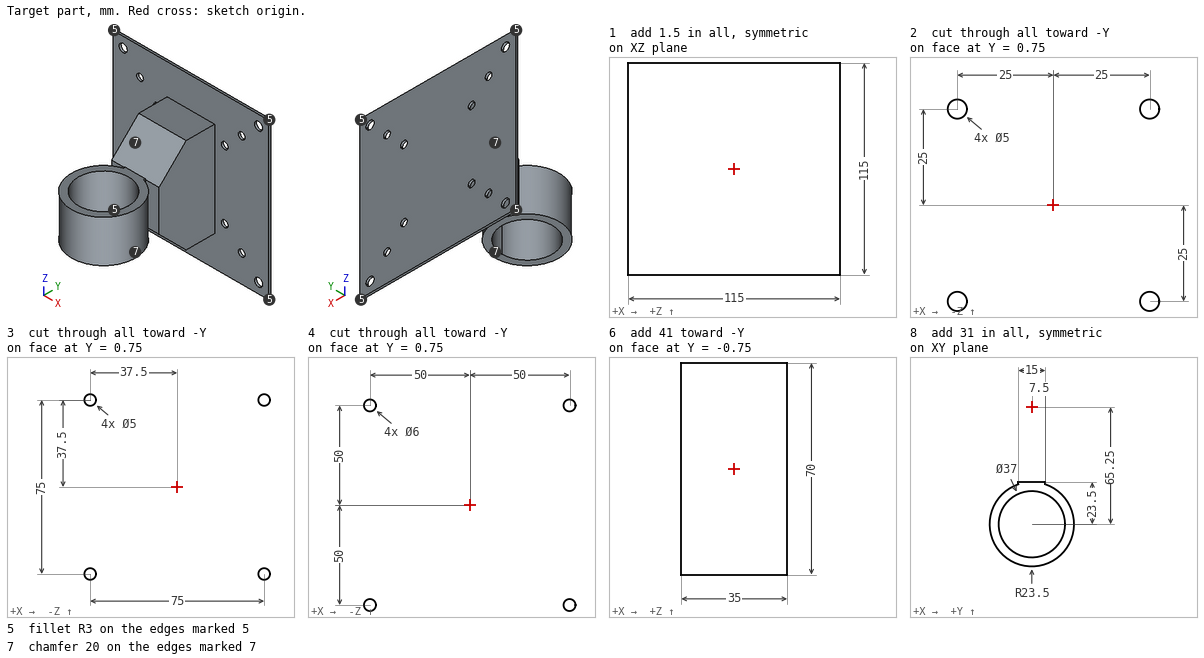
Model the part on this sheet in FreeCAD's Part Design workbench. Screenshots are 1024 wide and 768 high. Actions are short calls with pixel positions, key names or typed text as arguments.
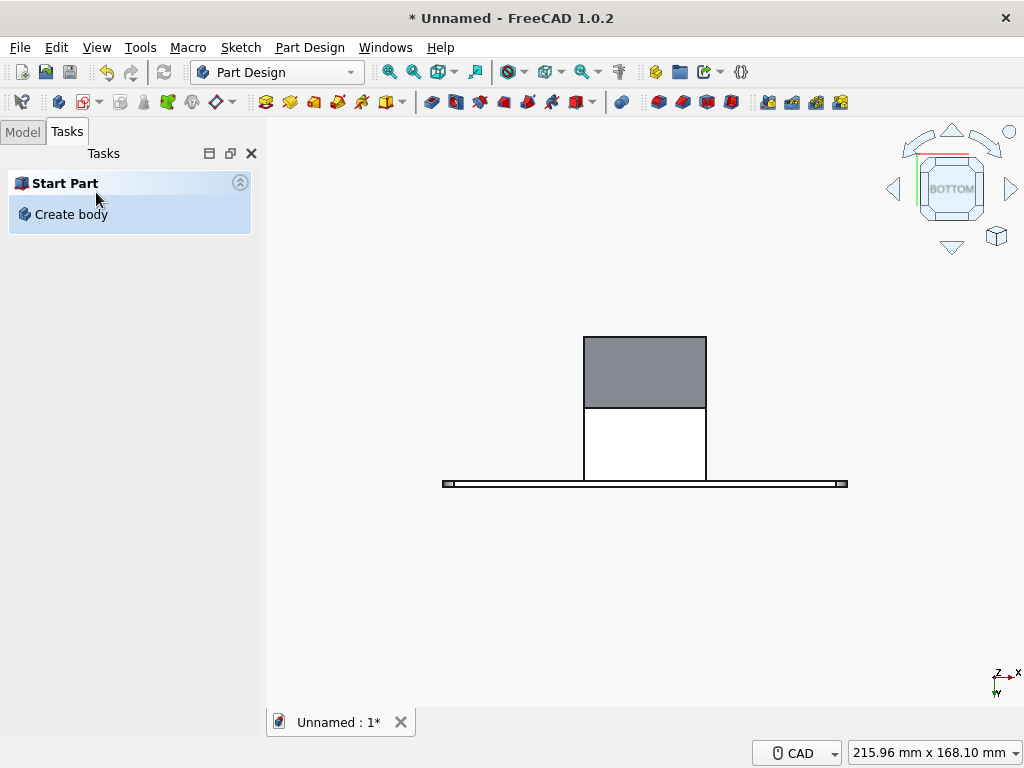
click(84, 102)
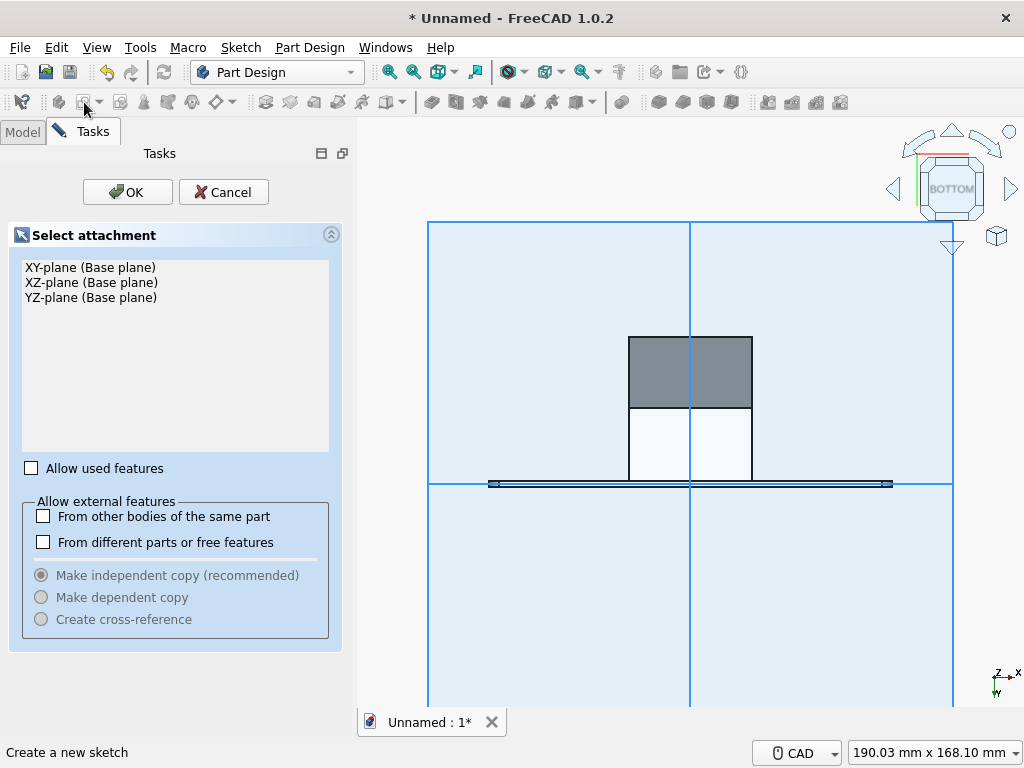
click(82, 268)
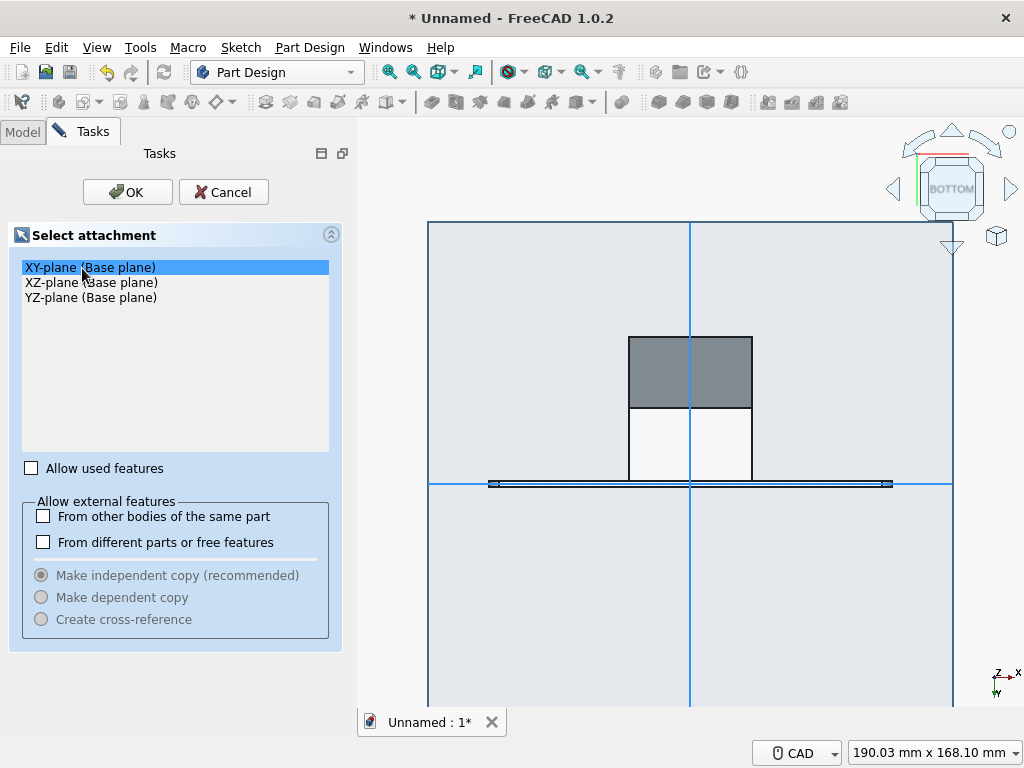
click(128, 192)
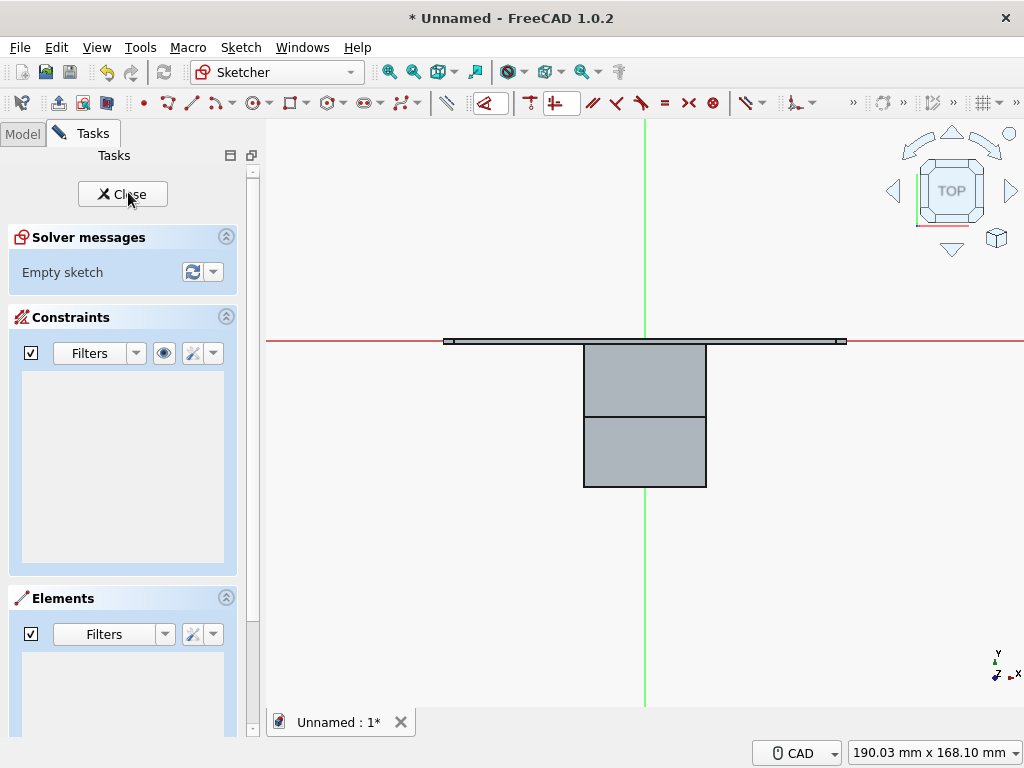
key(q)
key(s)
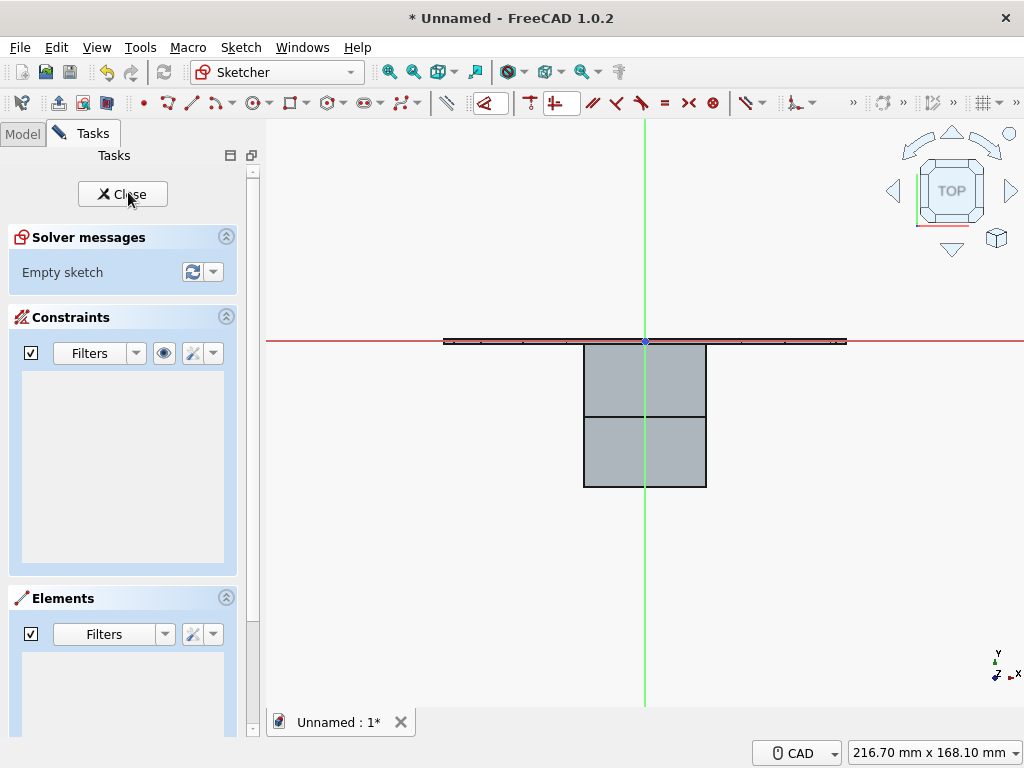
key(g)
key(m)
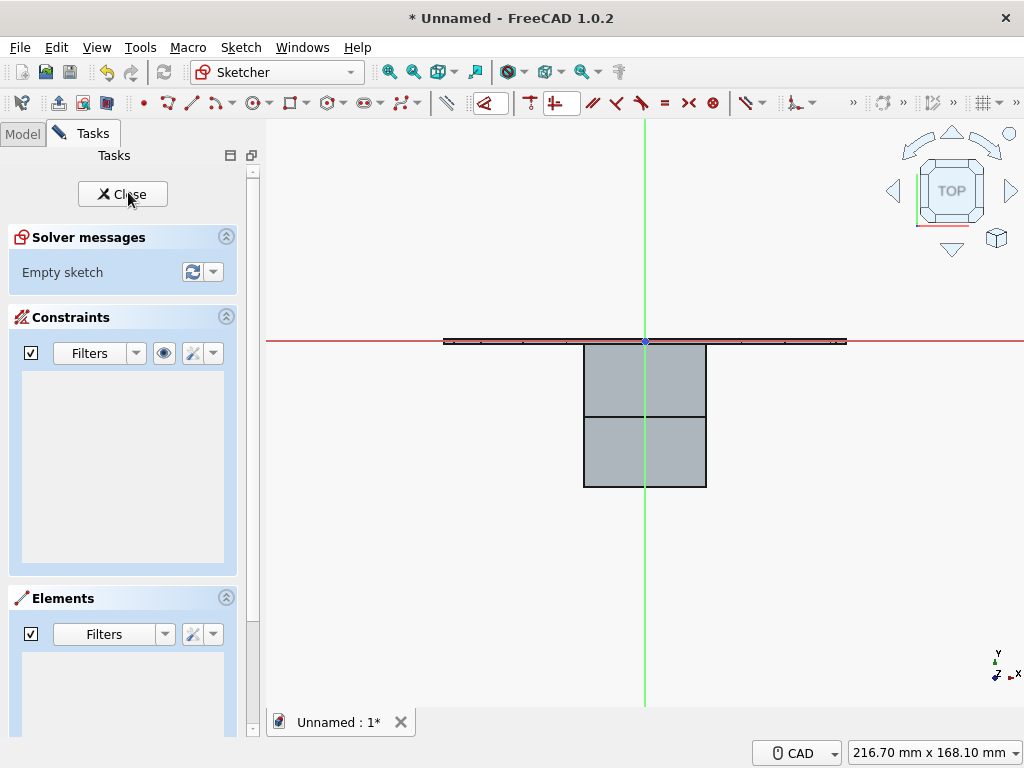
click(671, 492)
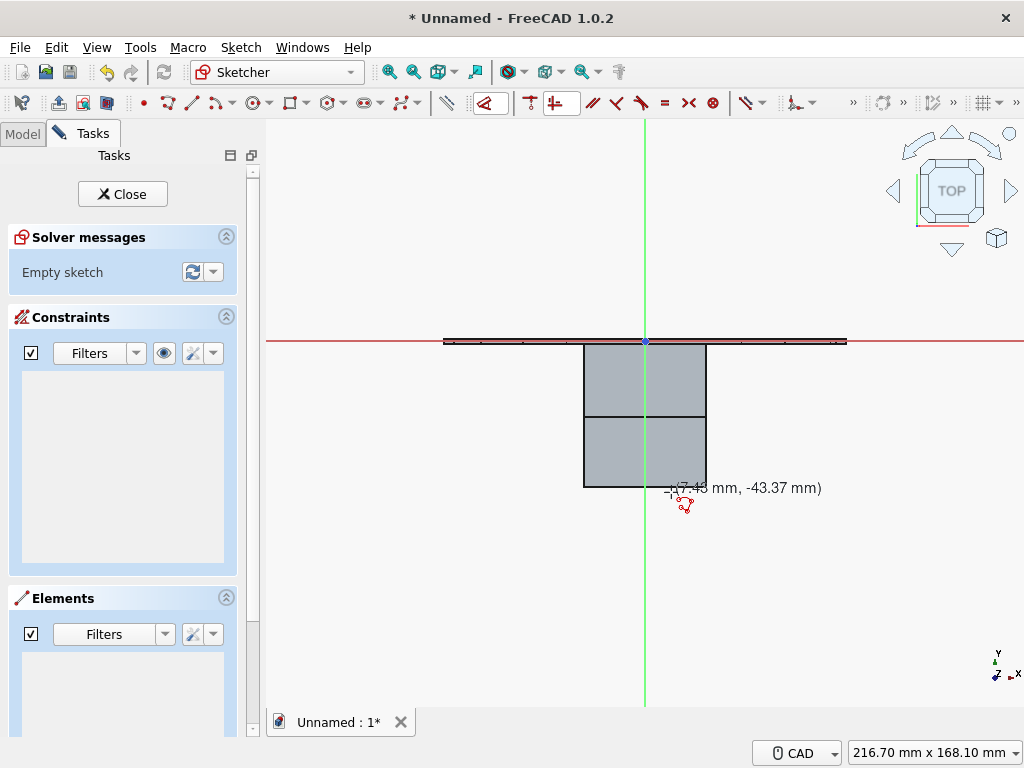
scroll(671, 487, up, 7)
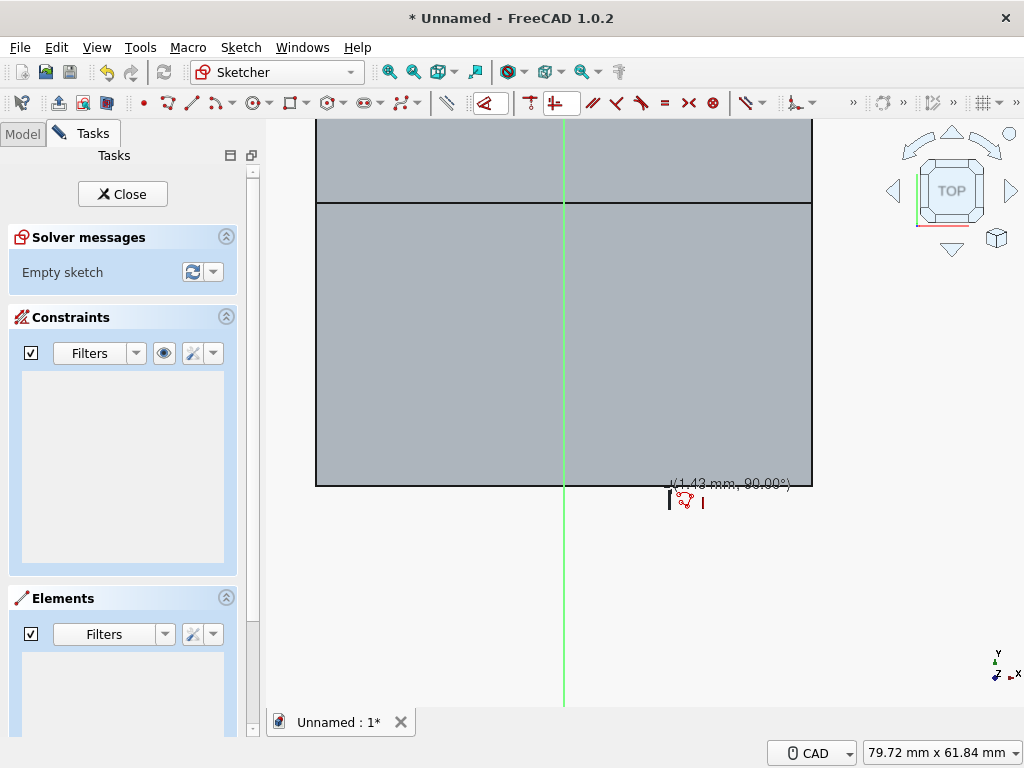
click(669, 486)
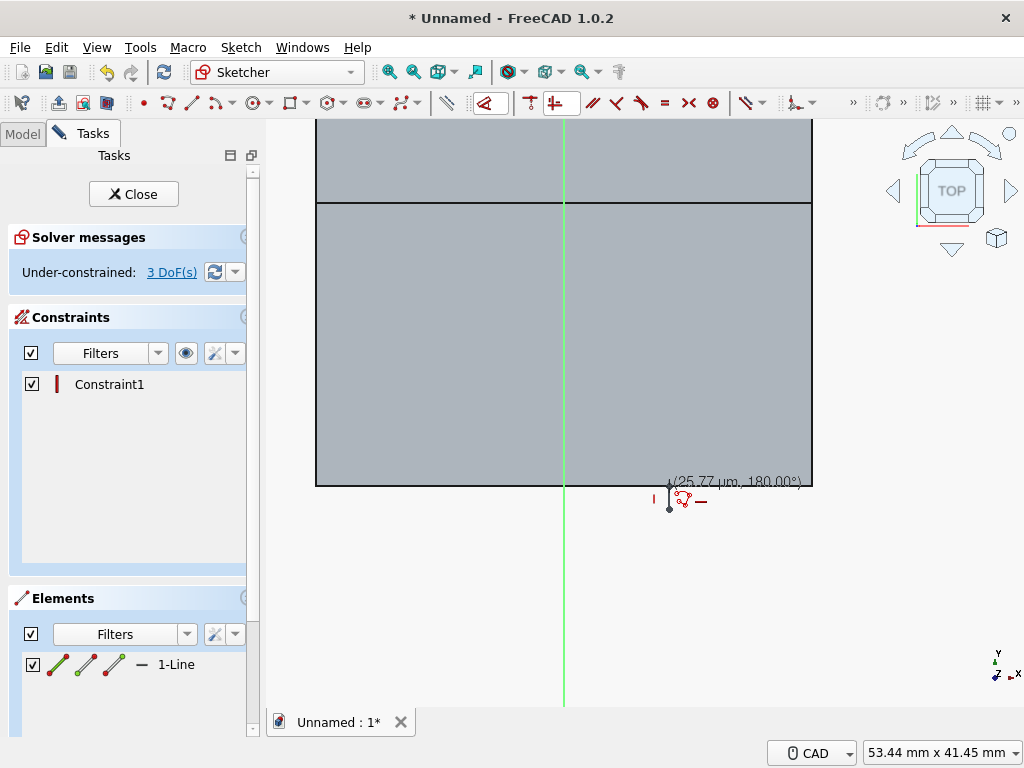
scroll(582, 365, down, 6)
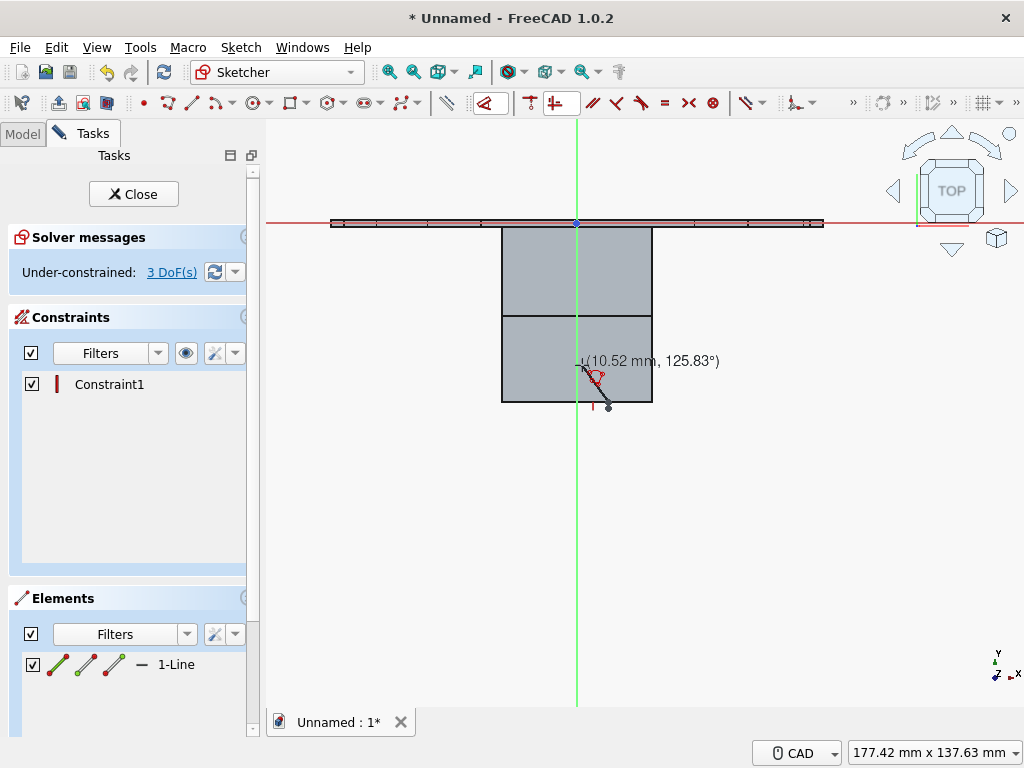
click(545, 402)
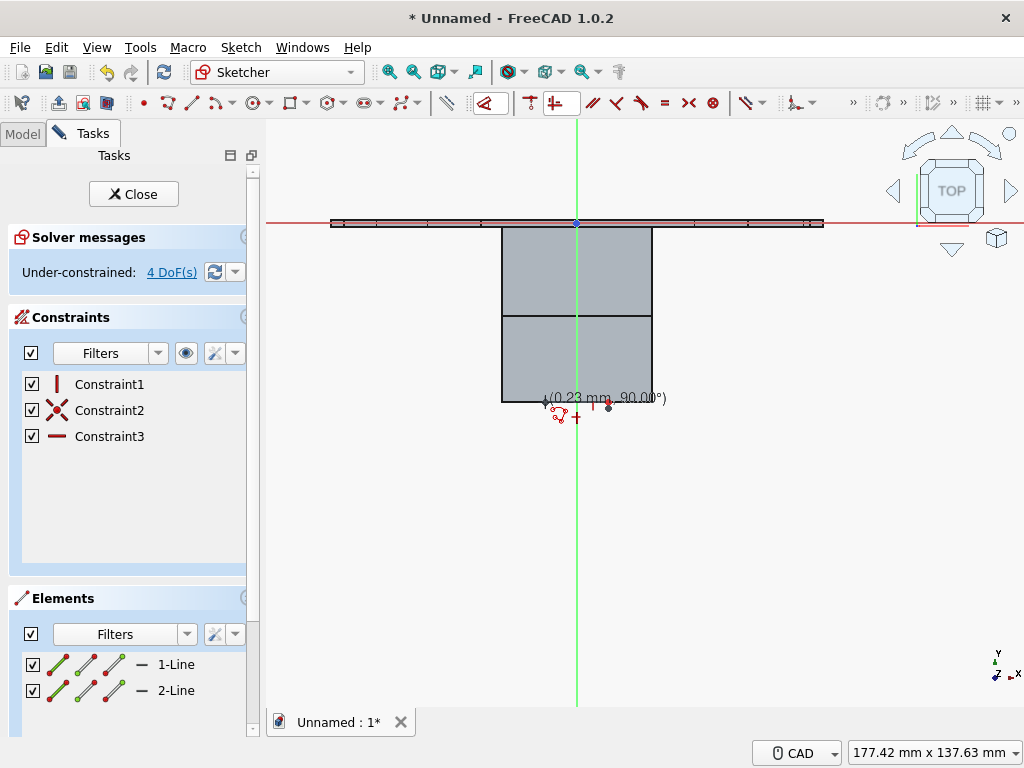
scroll(545, 407, up, 6)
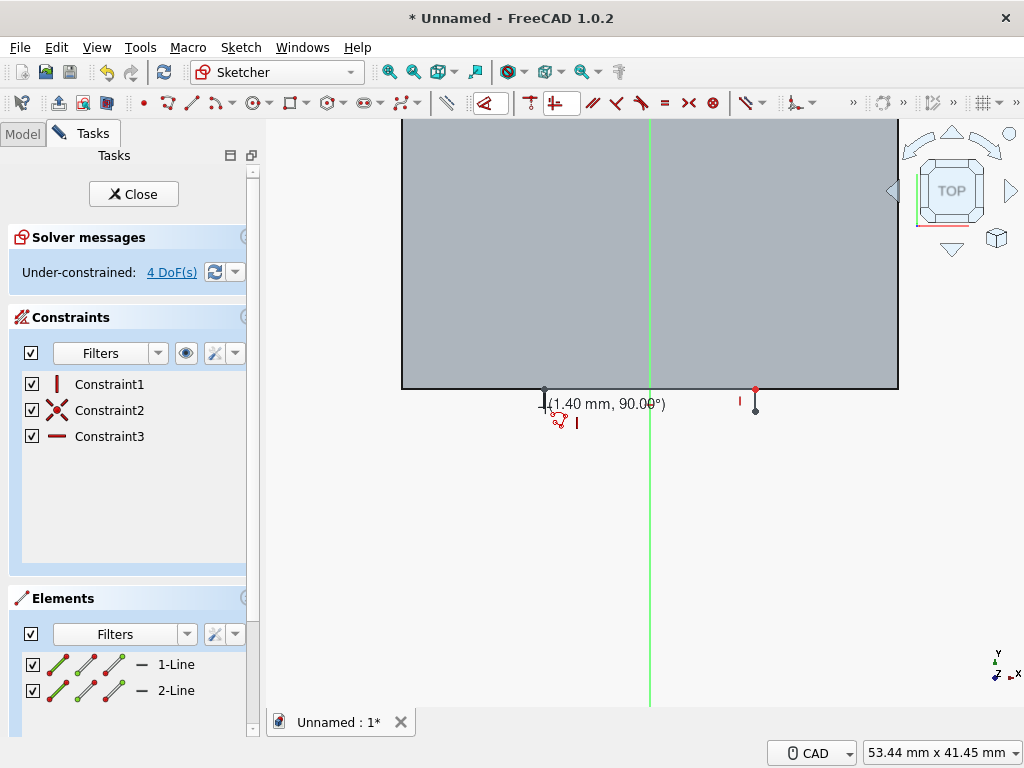
click(544, 406)
right_click(544, 406)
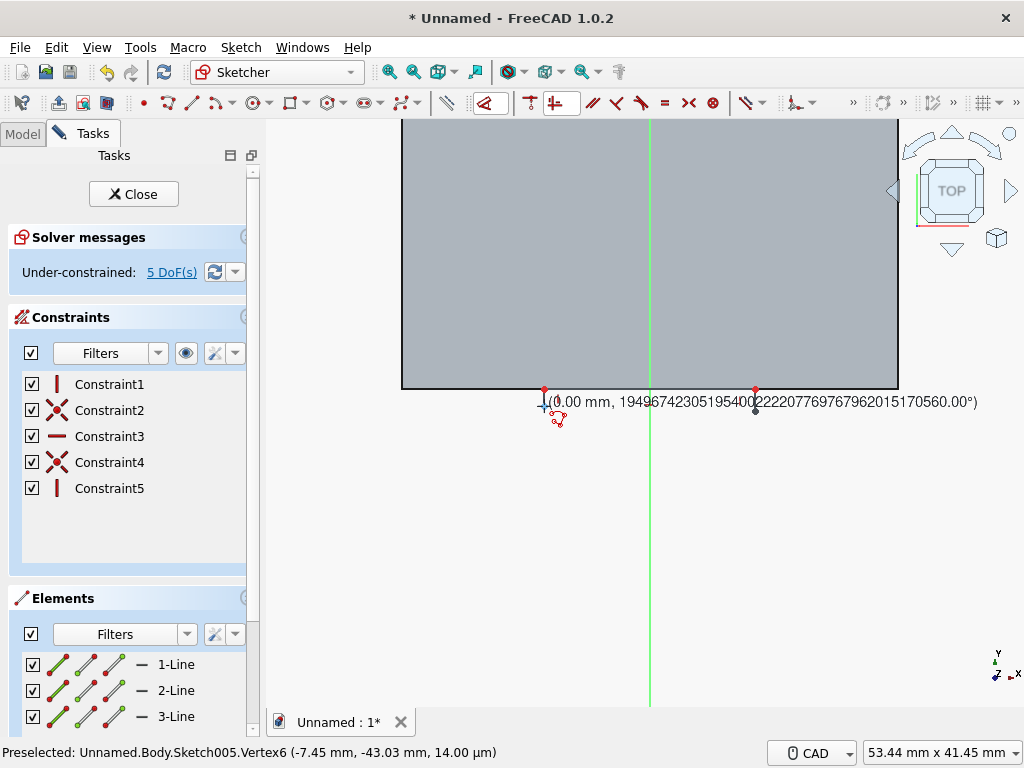
key(g)
key(3)
key(a)